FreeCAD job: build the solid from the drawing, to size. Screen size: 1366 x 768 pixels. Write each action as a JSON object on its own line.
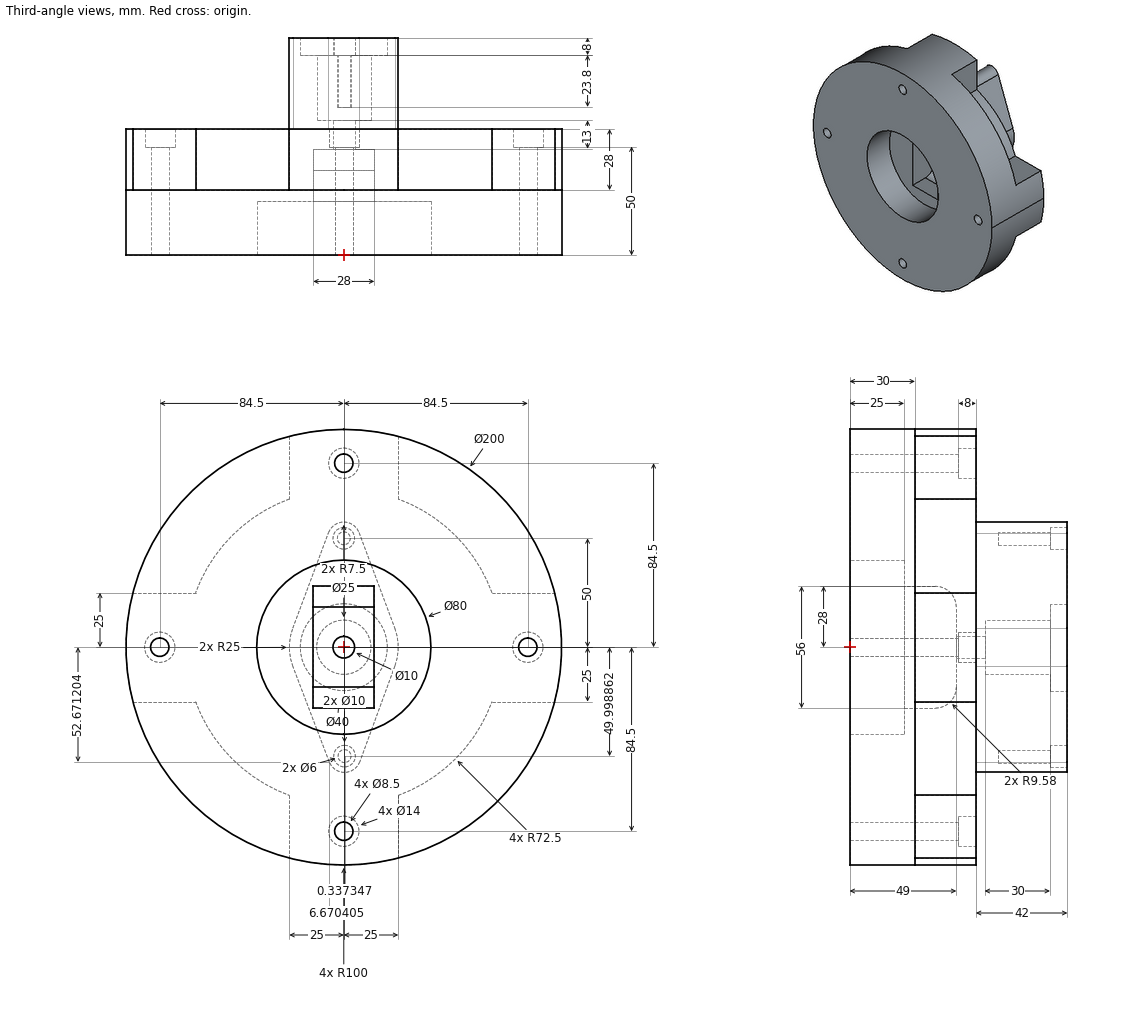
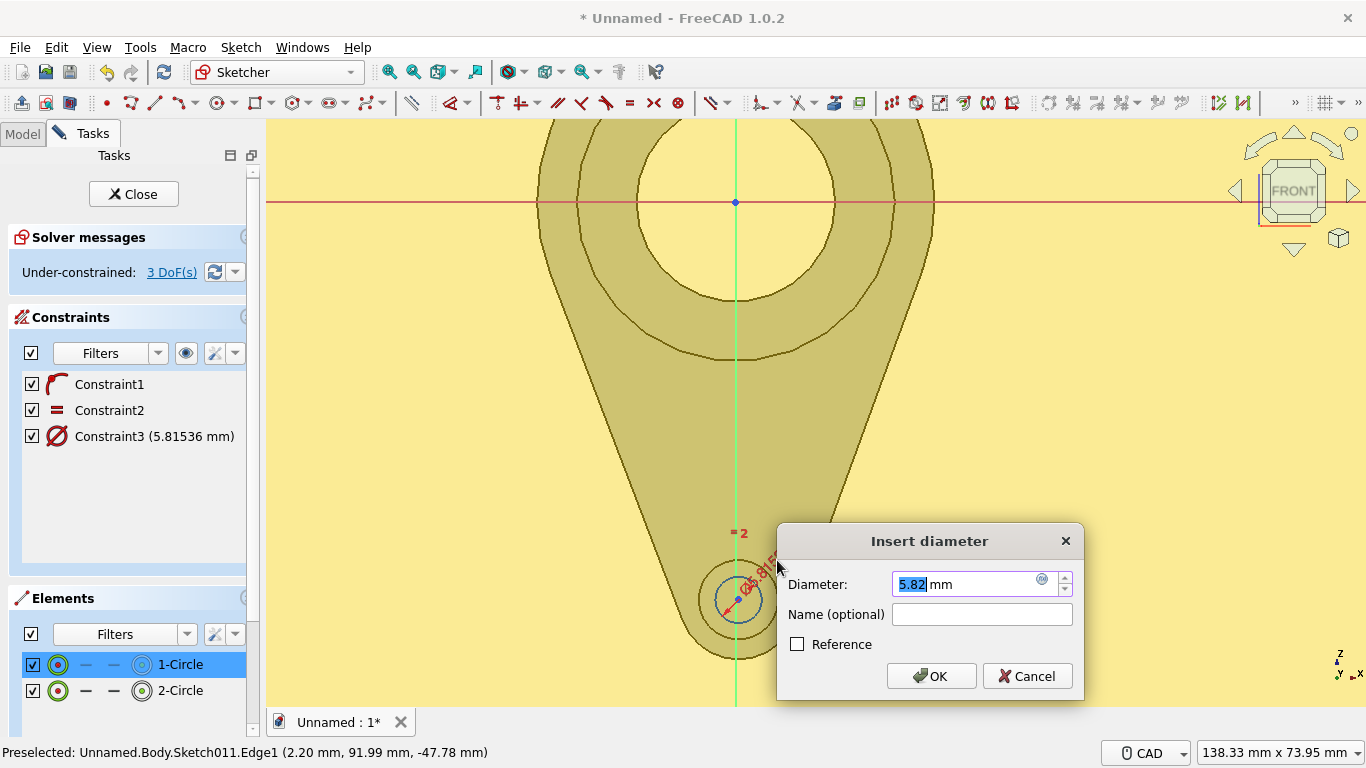
{"action": "type", "text": "6"}
{"action": "key", "text": "Return"}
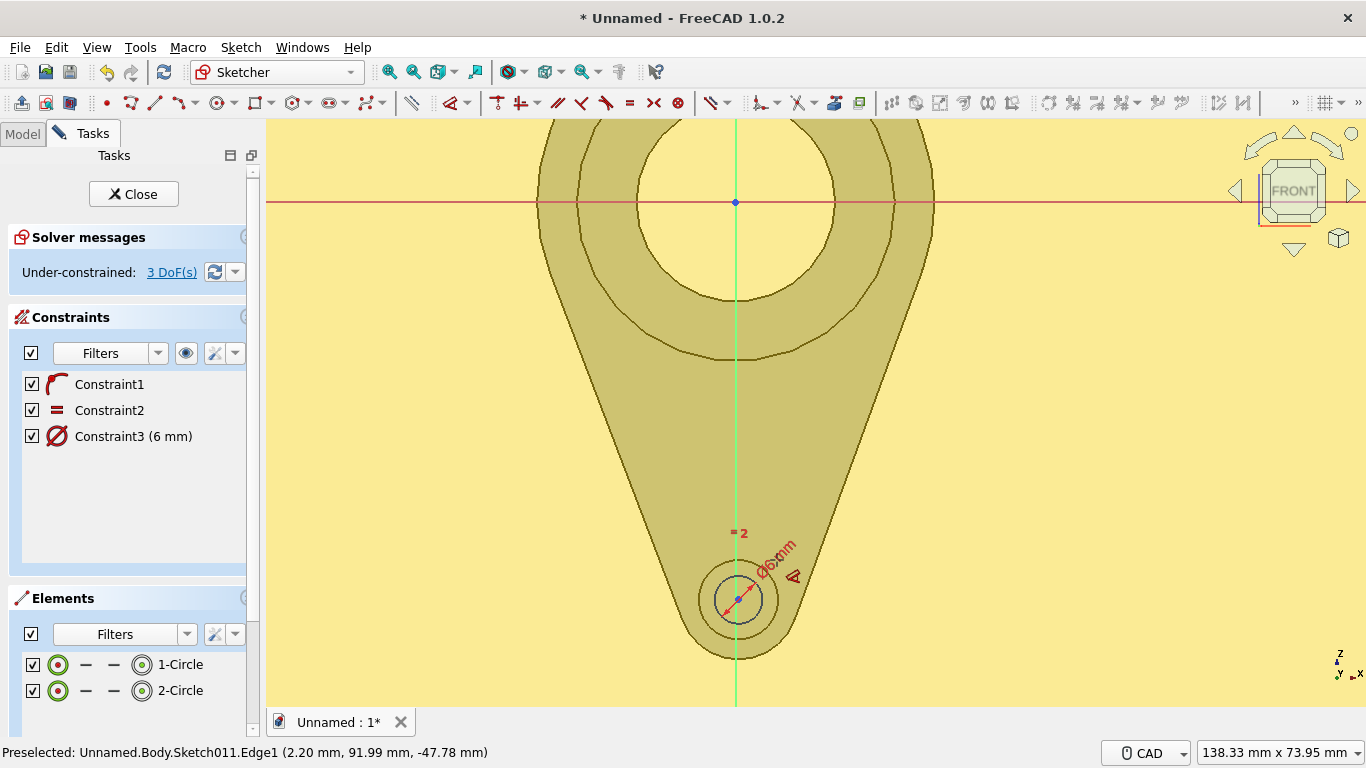
{"action": "scroll", "coordinate": [756, 585], "scroll_direction": "down", "scroll_amount": 4}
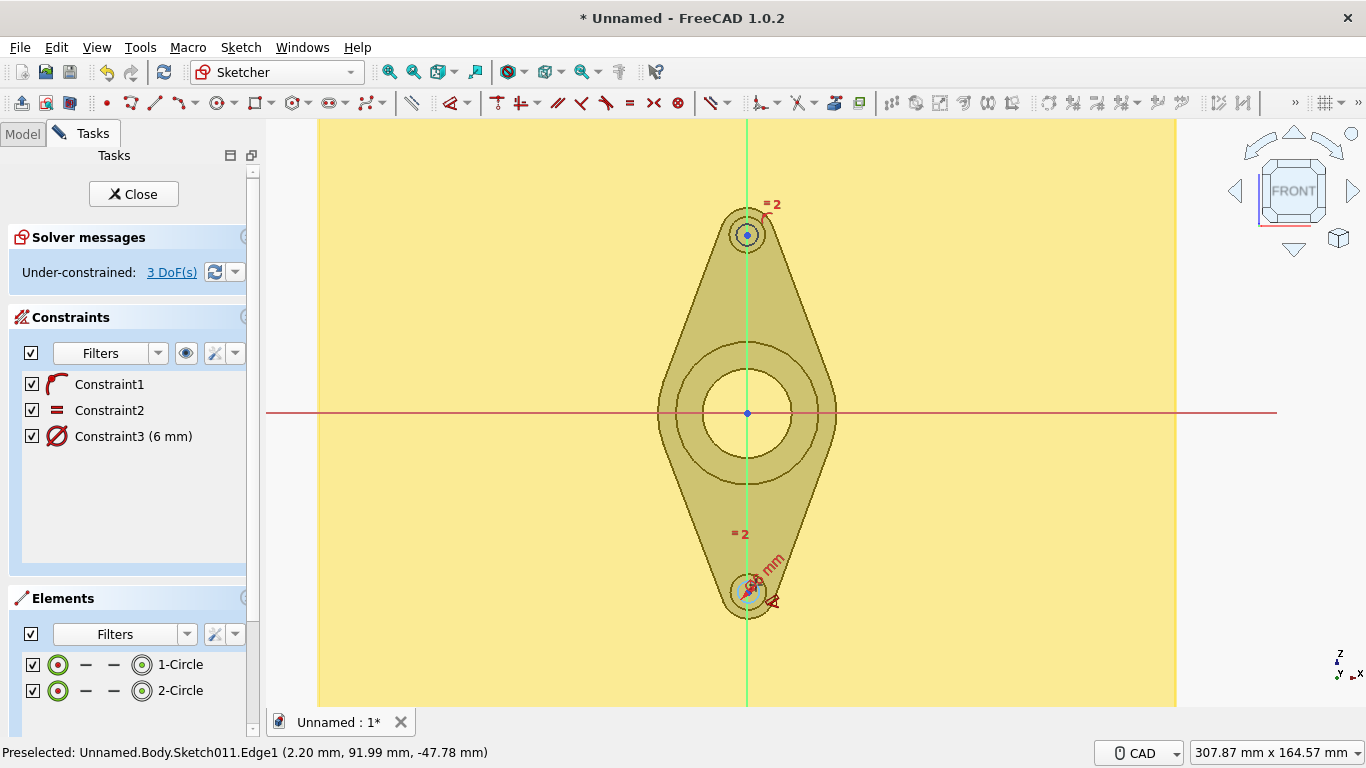
{"action": "left_click", "coordinate": [747, 235]}
{"action": "left_click", "coordinate": [713, 324]}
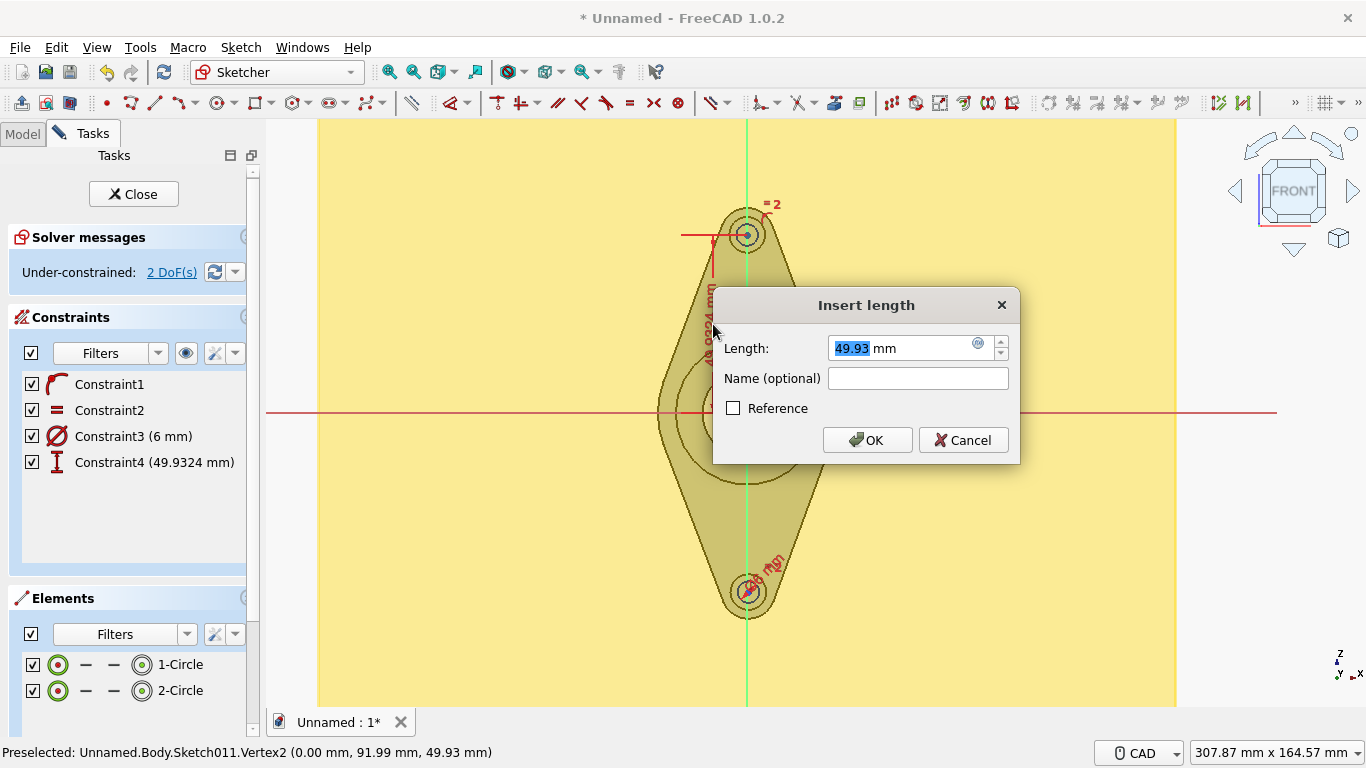
{"action": "type", "text": "50"}
{"action": "key", "text": "Return"}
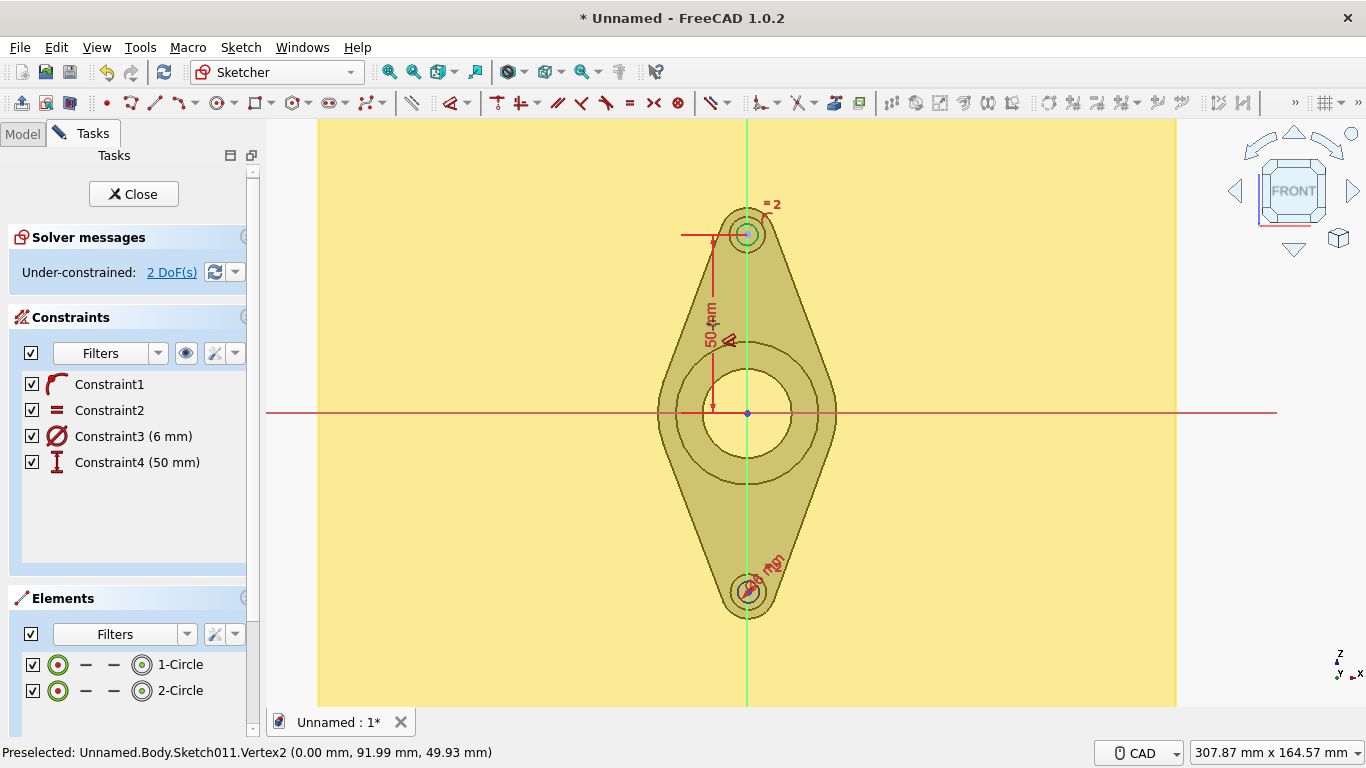
{"action": "scroll", "coordinate": [748, 592], "scroll_direction": "up", "scroll_amount": 18}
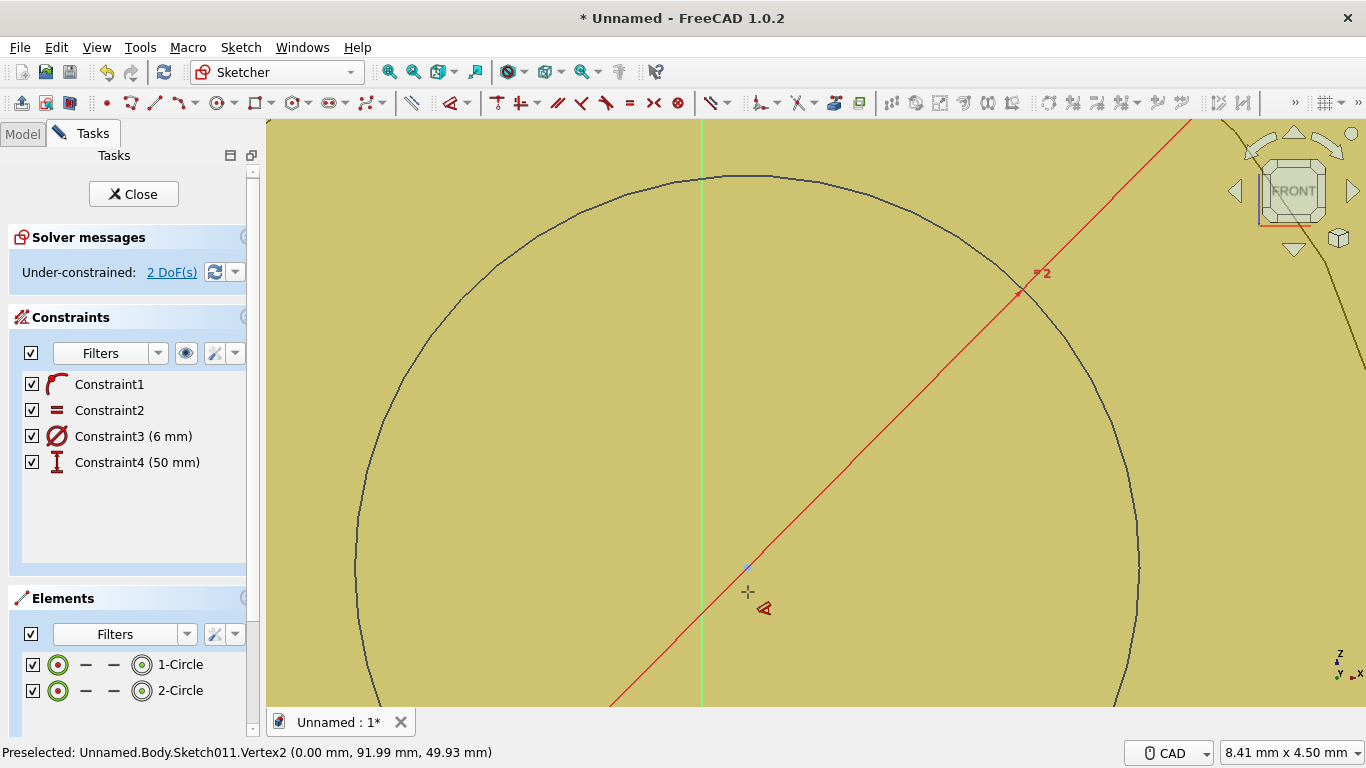
{"action": "left_click", "coordinate": [747, 568]}
{"action": "left_click", "coordinate": [725, 602]}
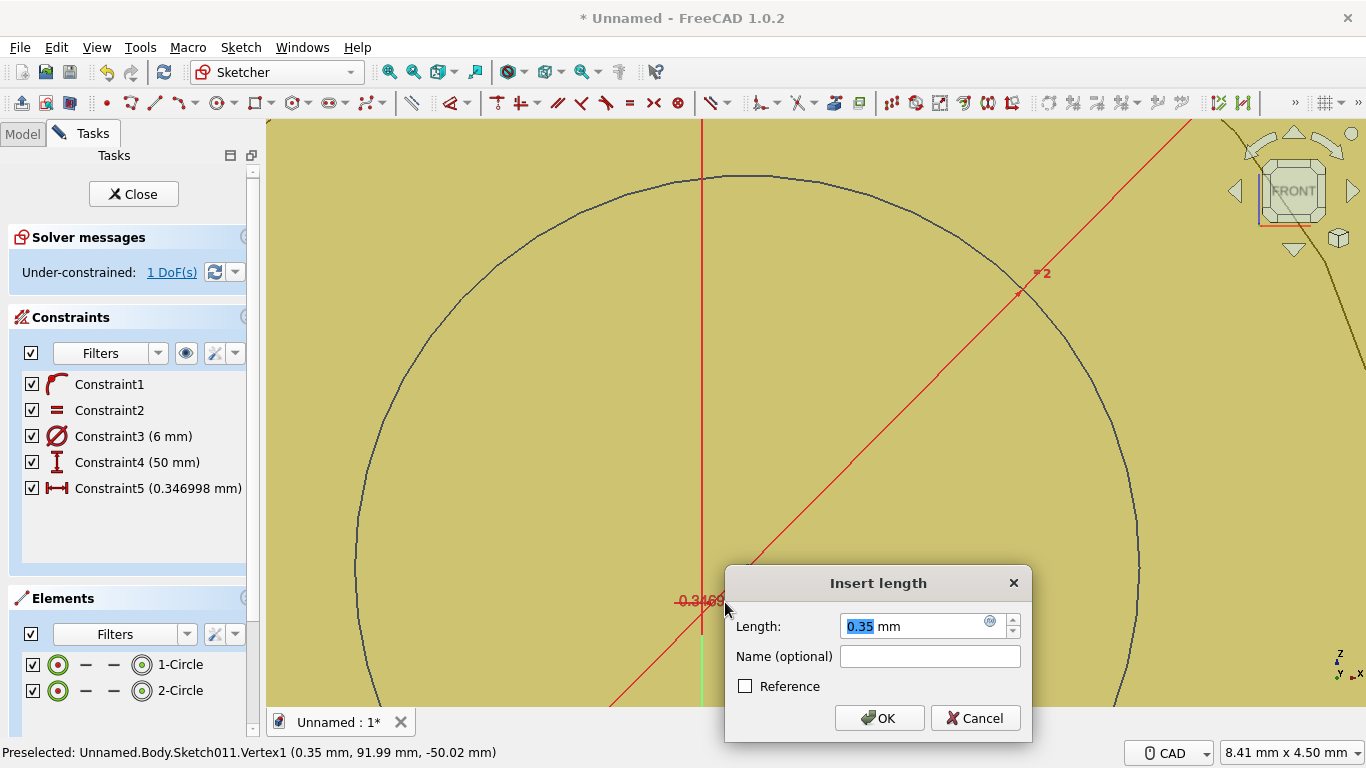
{"action": "type", "text": "0.337347"}
{"action": "key", "text": "Return"}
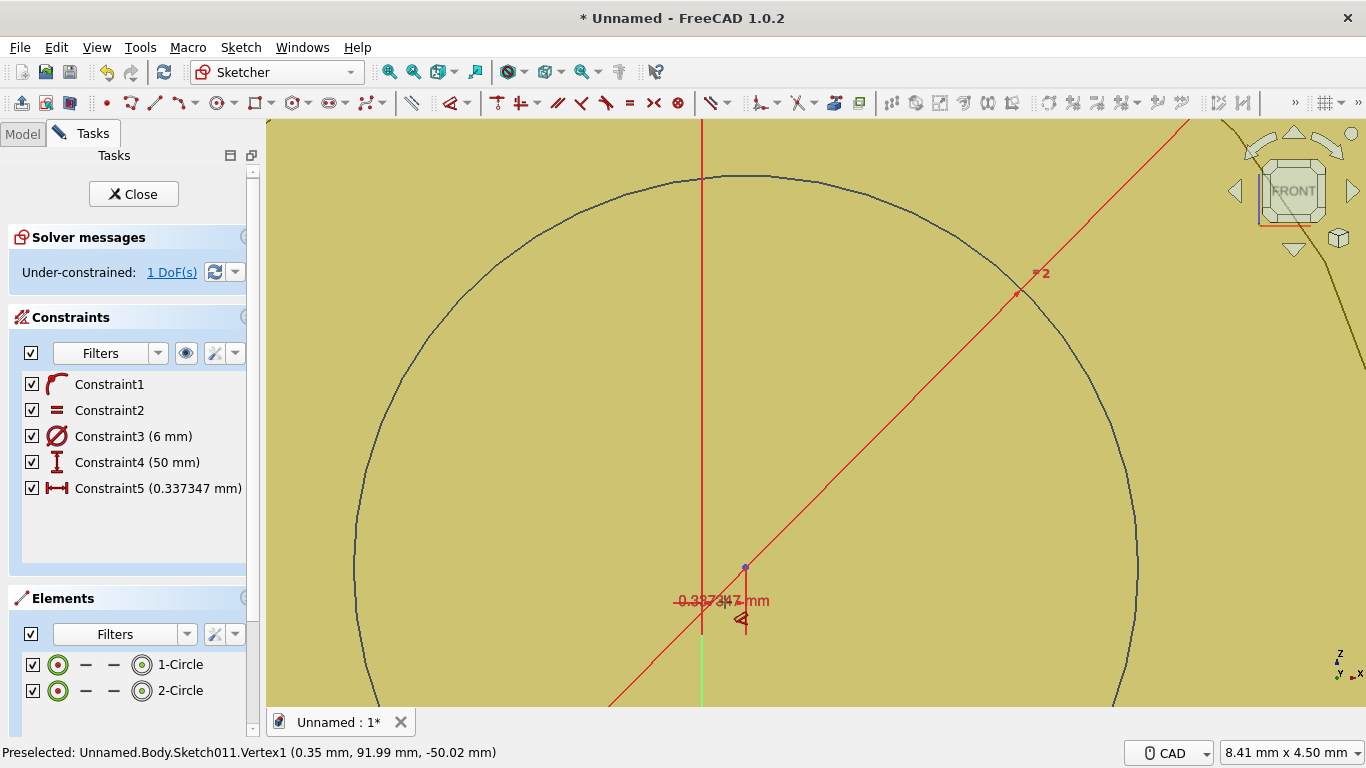
{"action": "scroll", "coordinate": [748, 633], "scroll_direction": "down", "scroll_amount": 17}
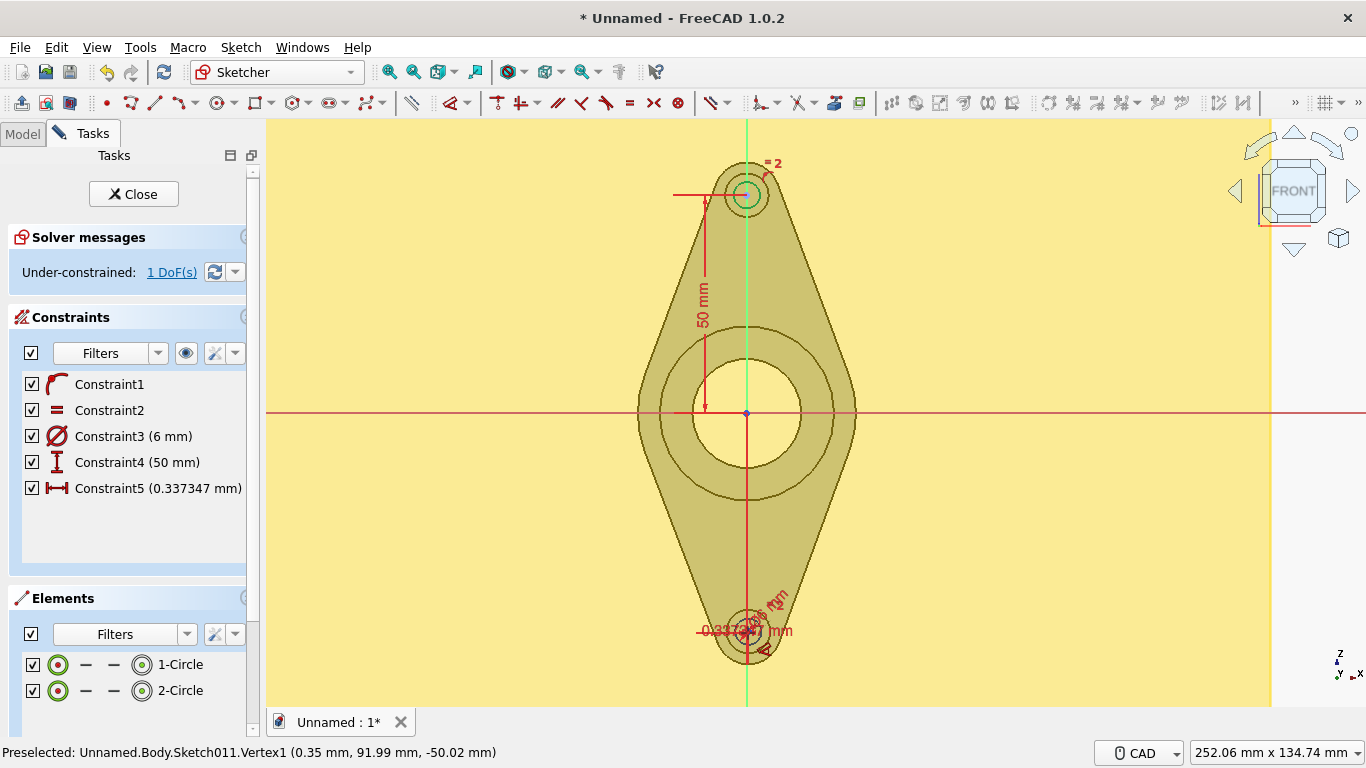
{"action": "left_click", "coordinate": [748, 632]}
{"action": "left_click", "coordinate": [713, 523]}